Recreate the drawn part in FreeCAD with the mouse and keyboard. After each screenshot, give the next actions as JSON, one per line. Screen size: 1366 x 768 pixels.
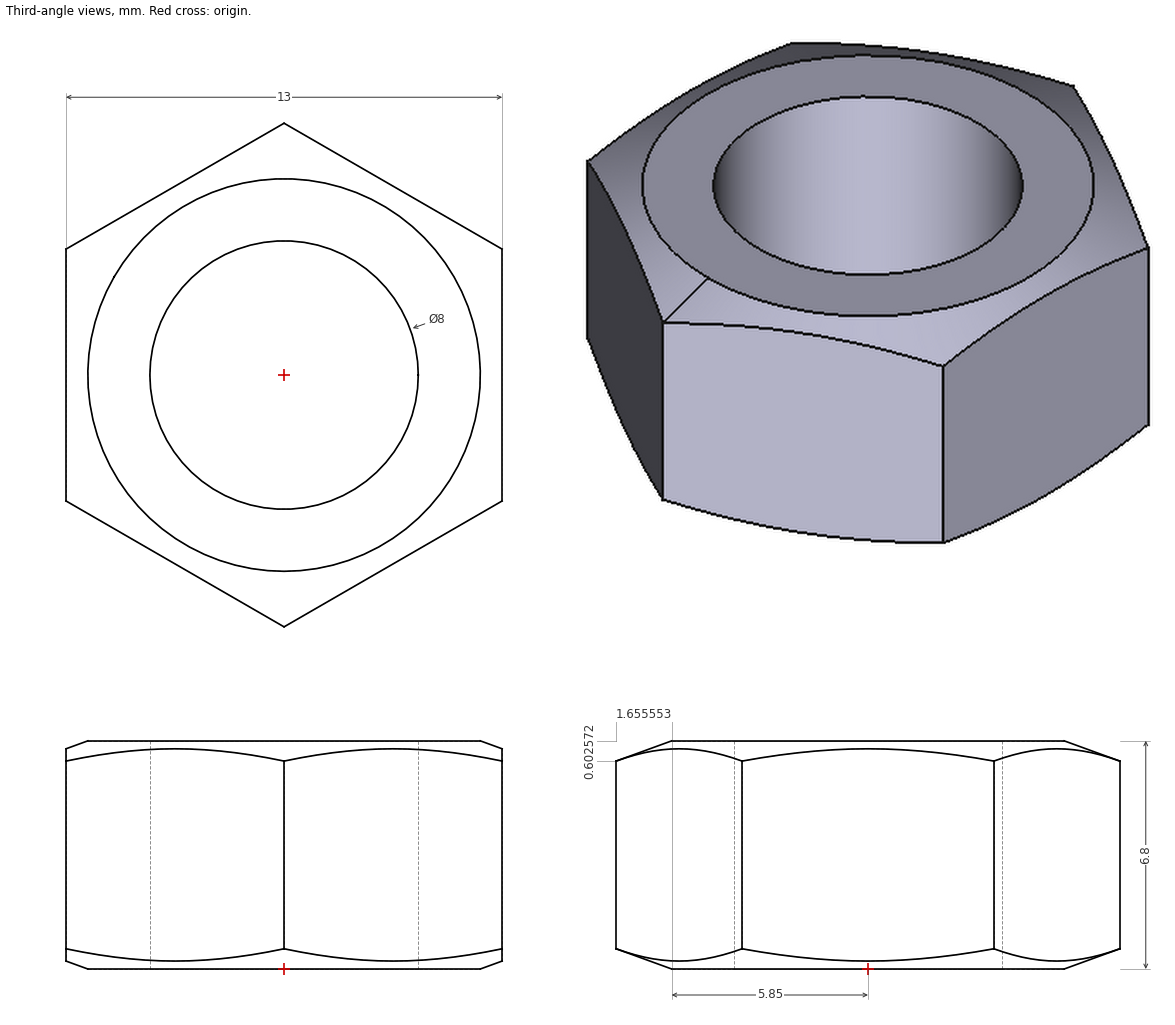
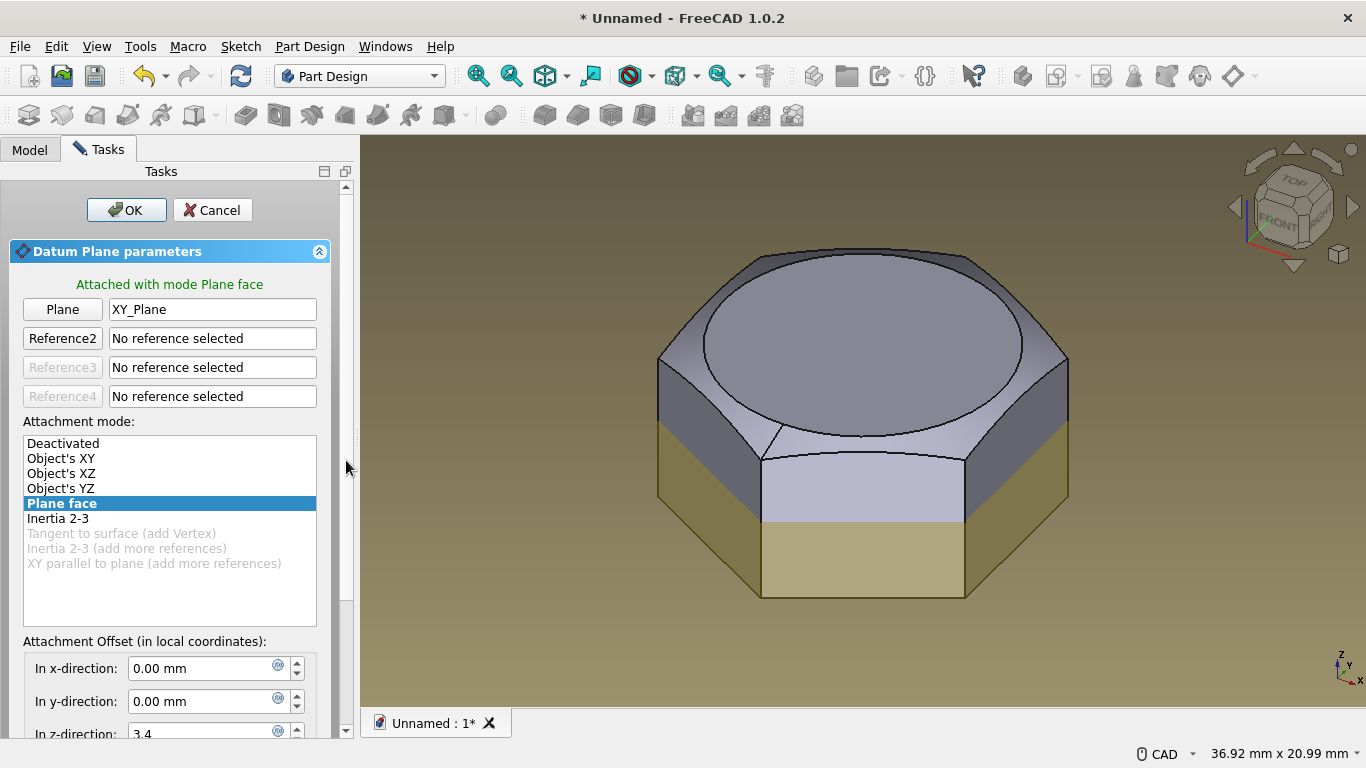
{"action": "left_click", "coordinate": [127, 210]}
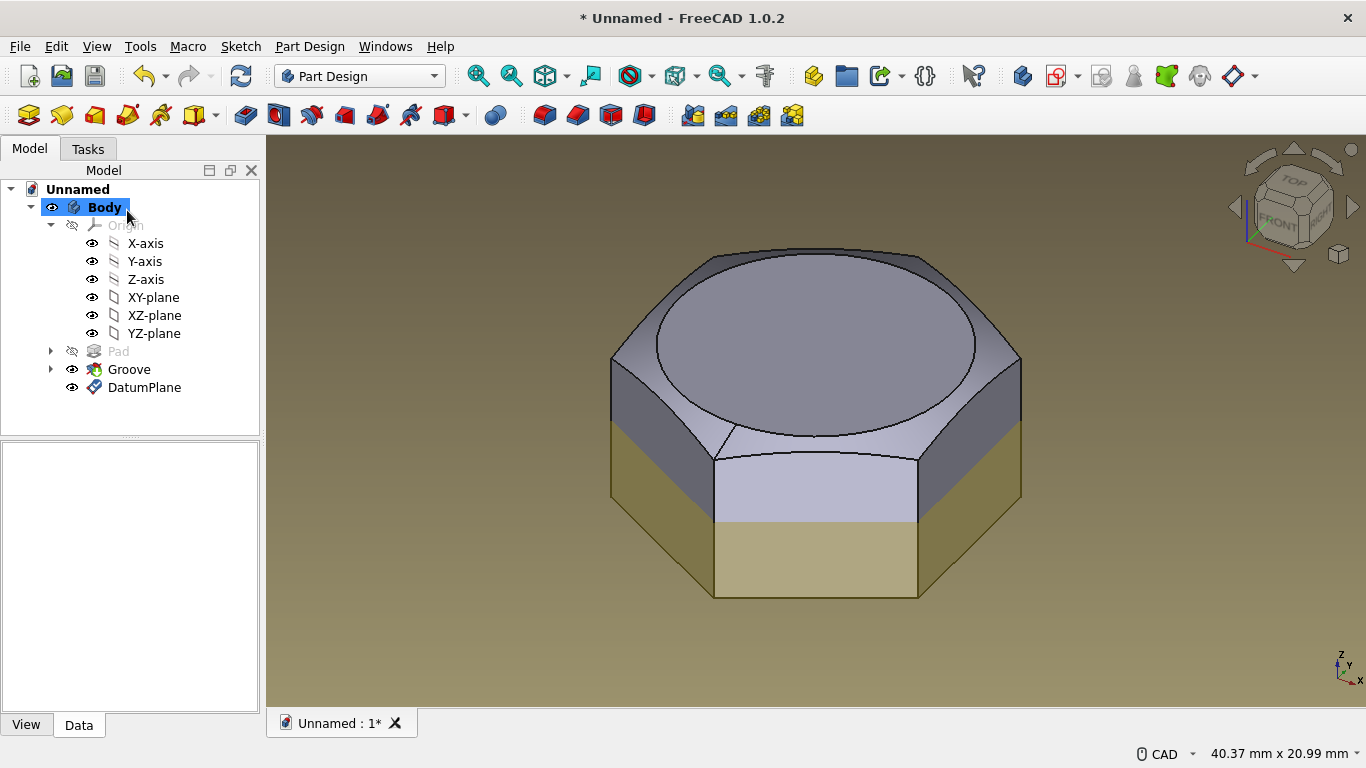
{"action": "left_click", "coordinate": [117, 369]}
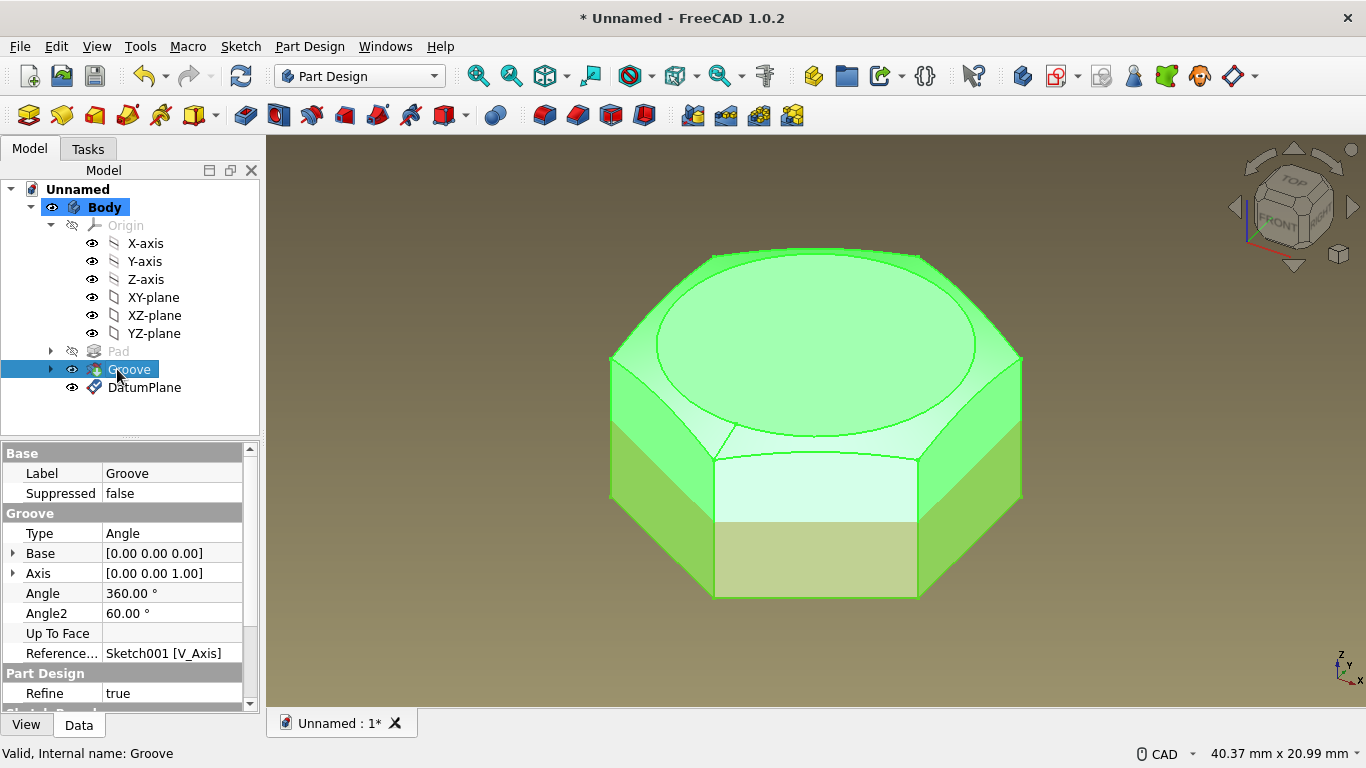
{"action": "left_click", "coordinate": [693, 116]}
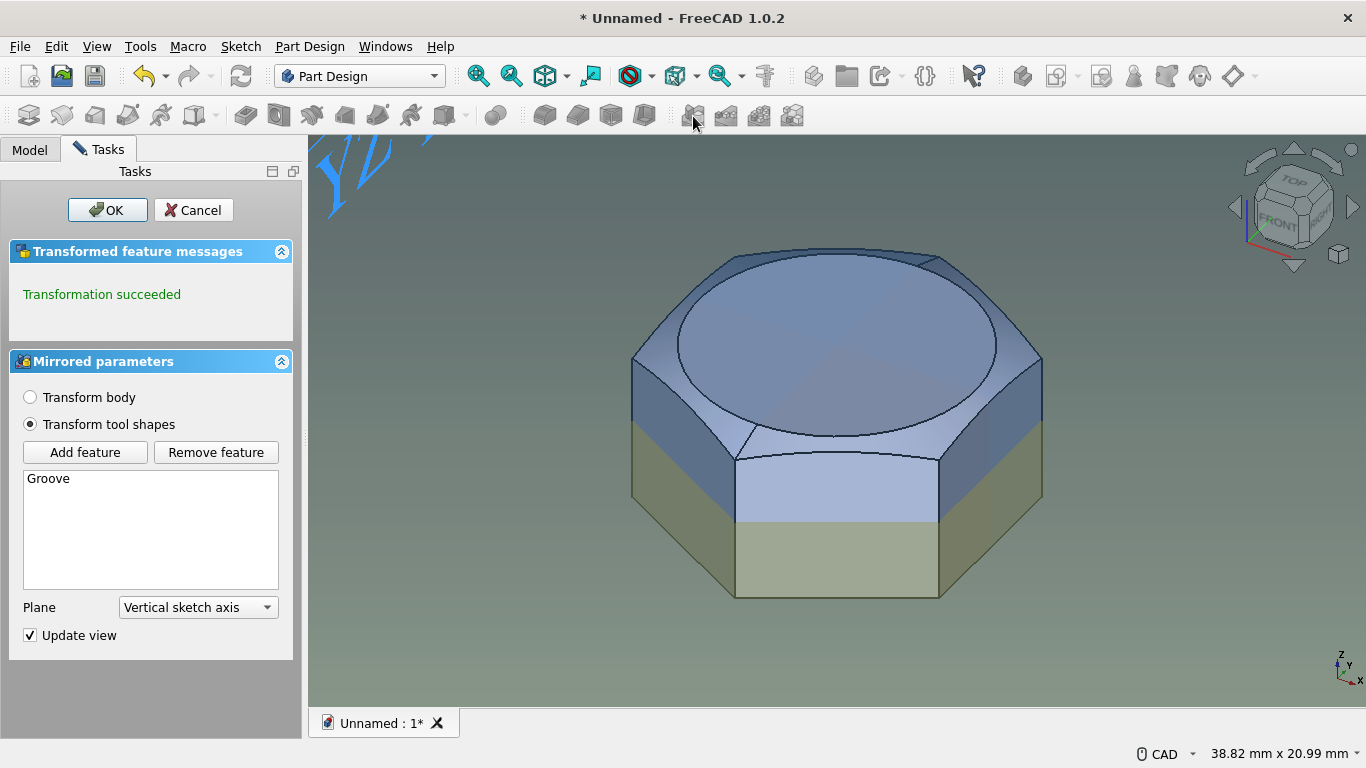
{"action": "left_click", "coordinate": [199, 608]}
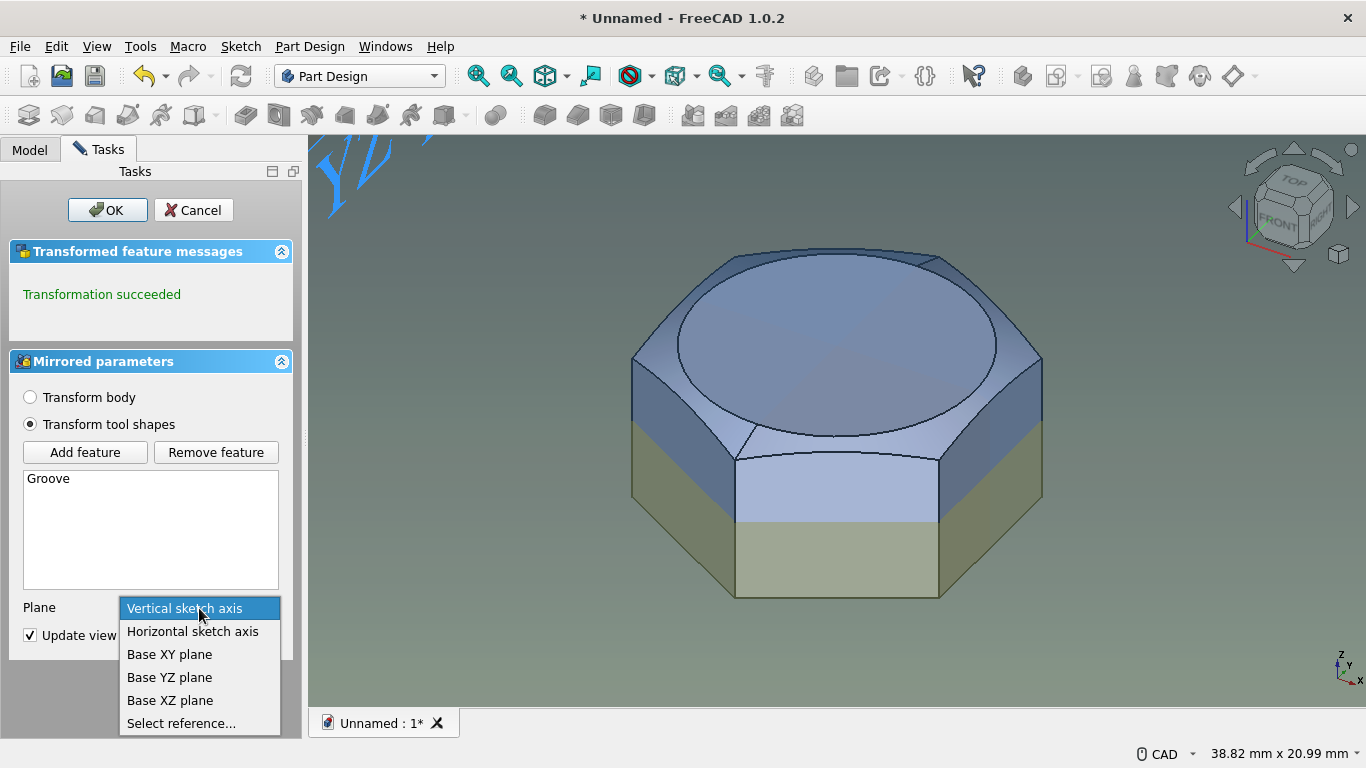
{"action": "left_click", "coordinate": [198, 724]}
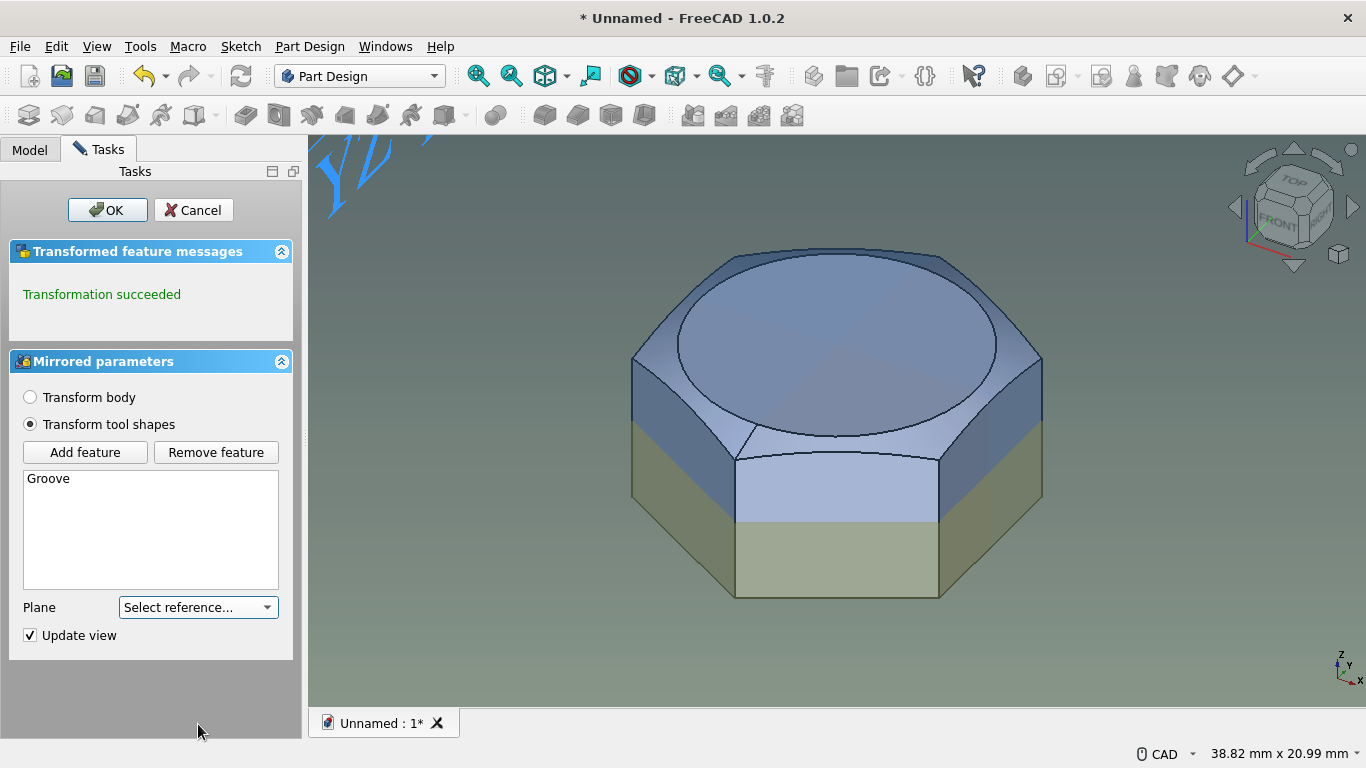
{"action": "left_click", "coordinate": [30, 149]}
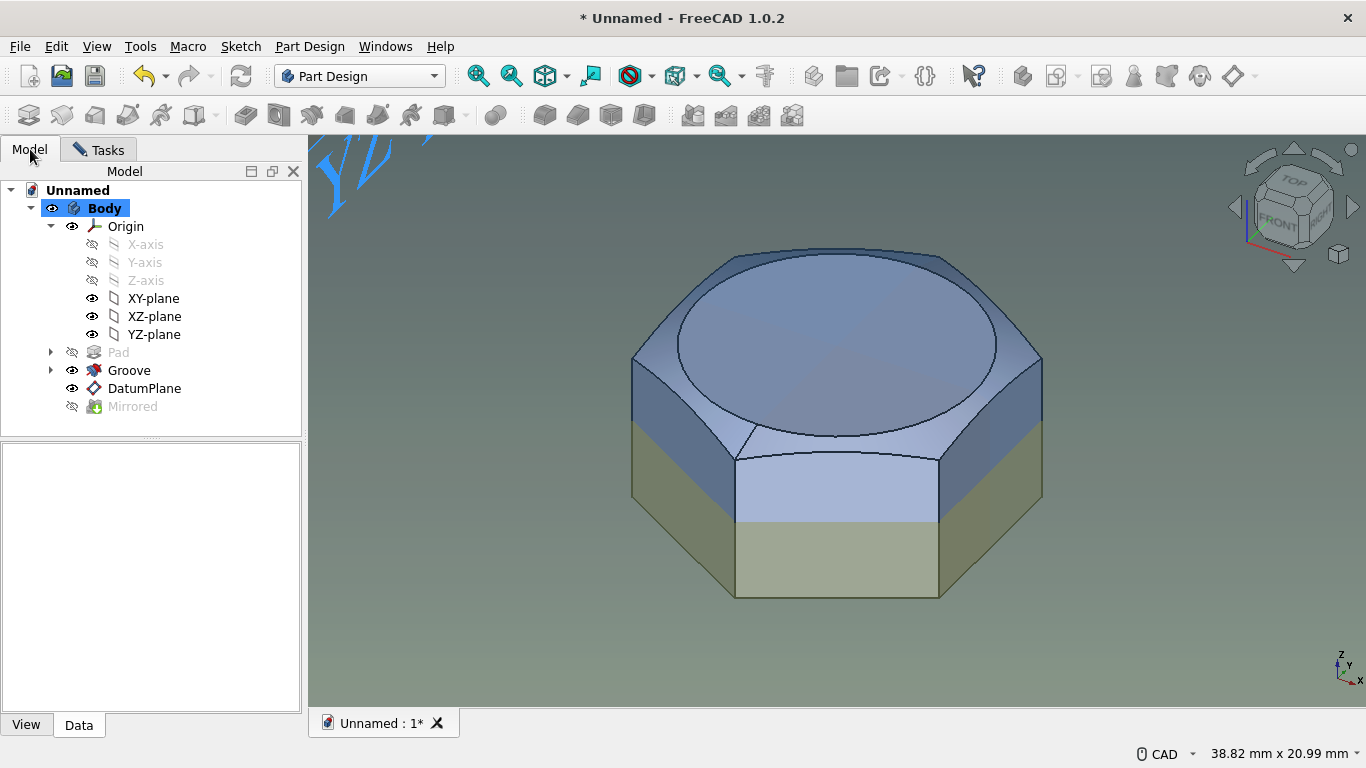
{"action": "left_click", "coordinate": [117, 388]}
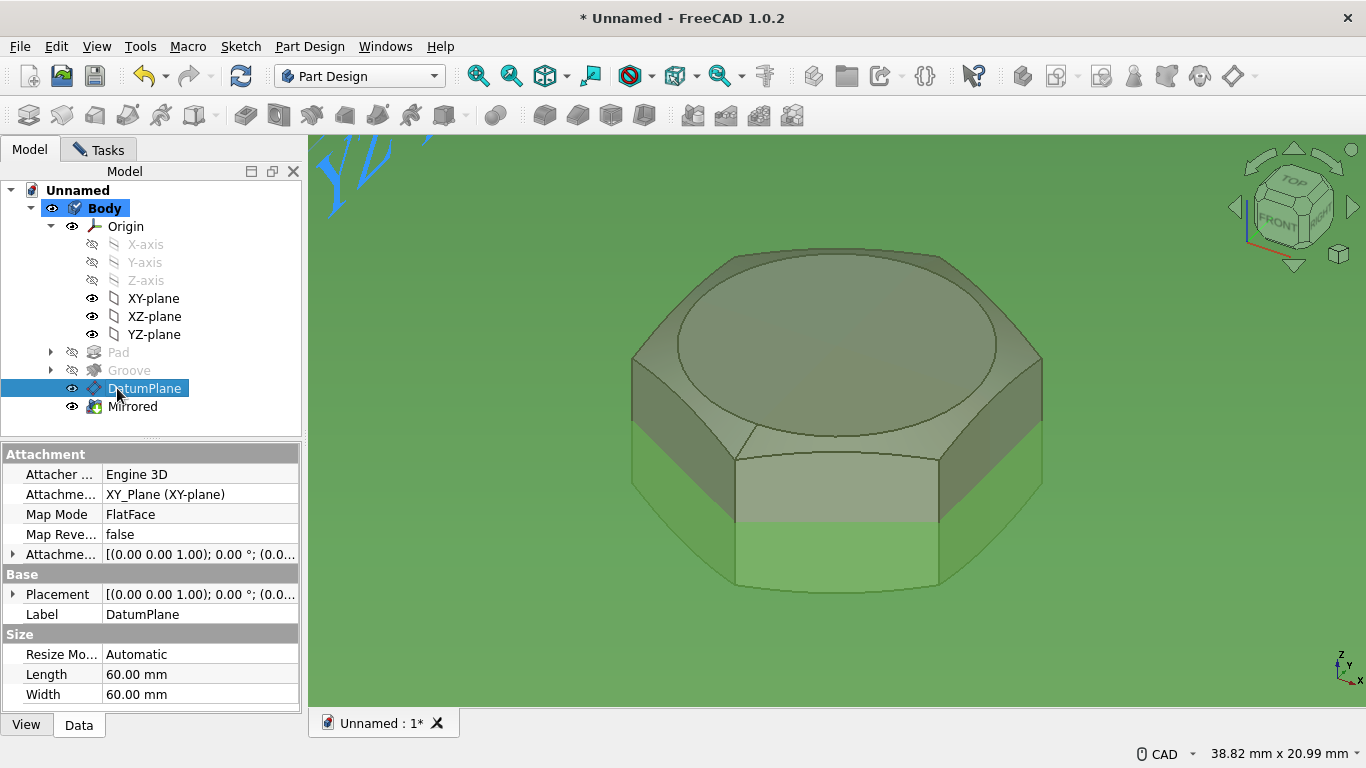
{"action": "left_click", "coordinate": [98, 149]}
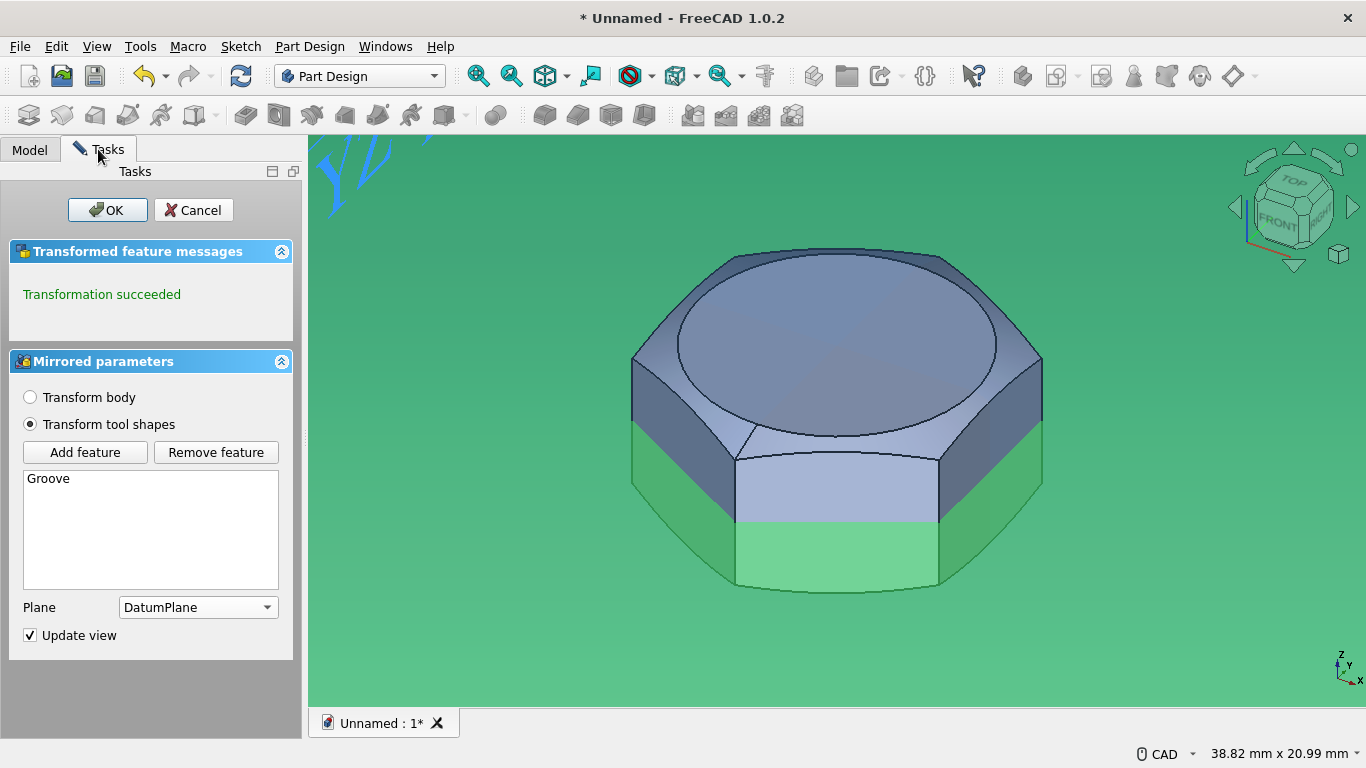
{"action": "left_click", "coordinate": [108, 210]}